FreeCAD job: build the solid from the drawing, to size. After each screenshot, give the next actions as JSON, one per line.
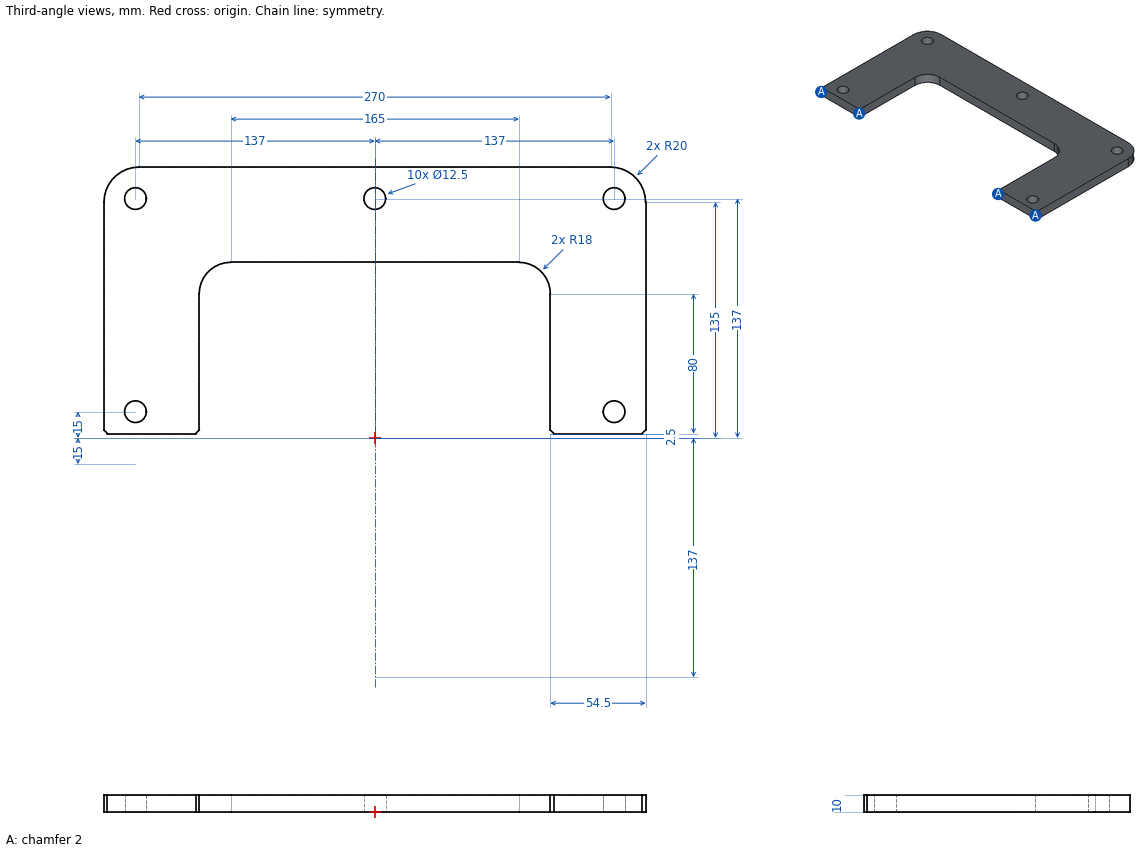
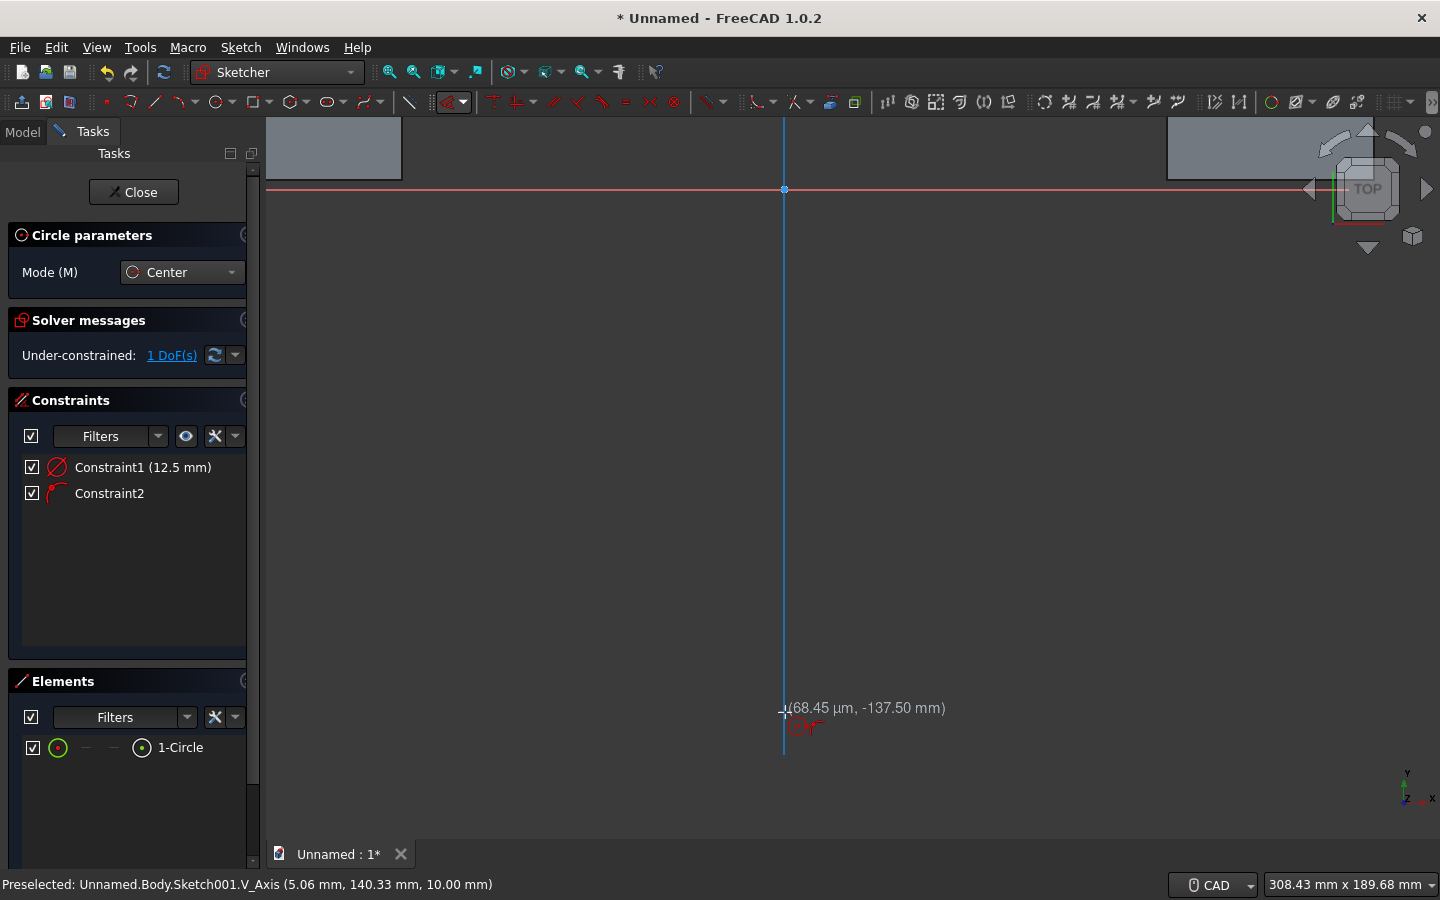
{"action": "left_click", "coordinate": [784, 711]}
{"action": "mouse_move", "coordinate": [801, 694]}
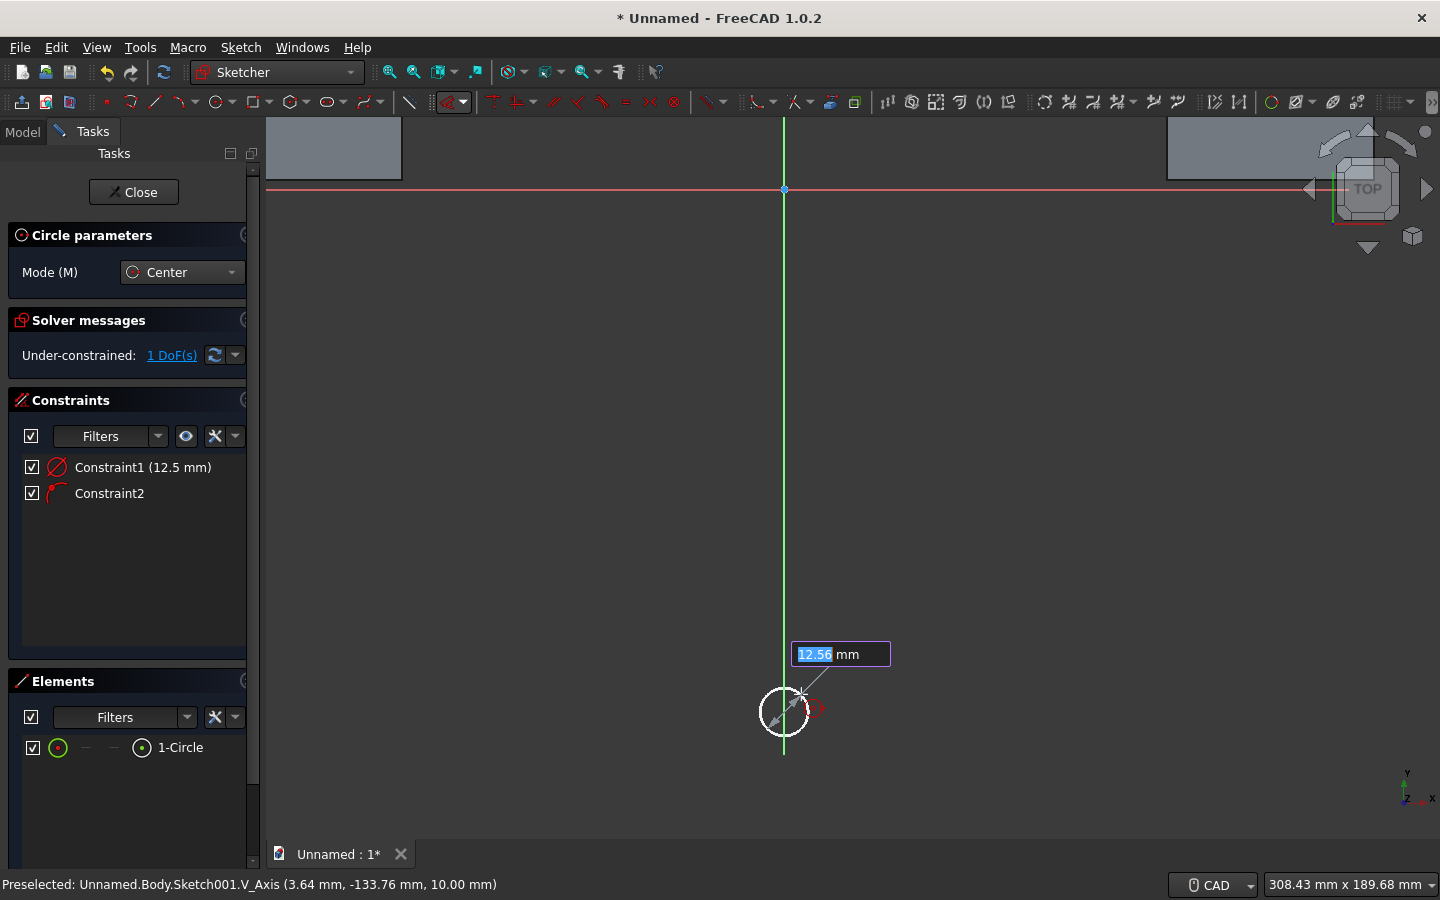
{"action": "type", "text": "12.5"}
{"action": "key", "text": "Return"}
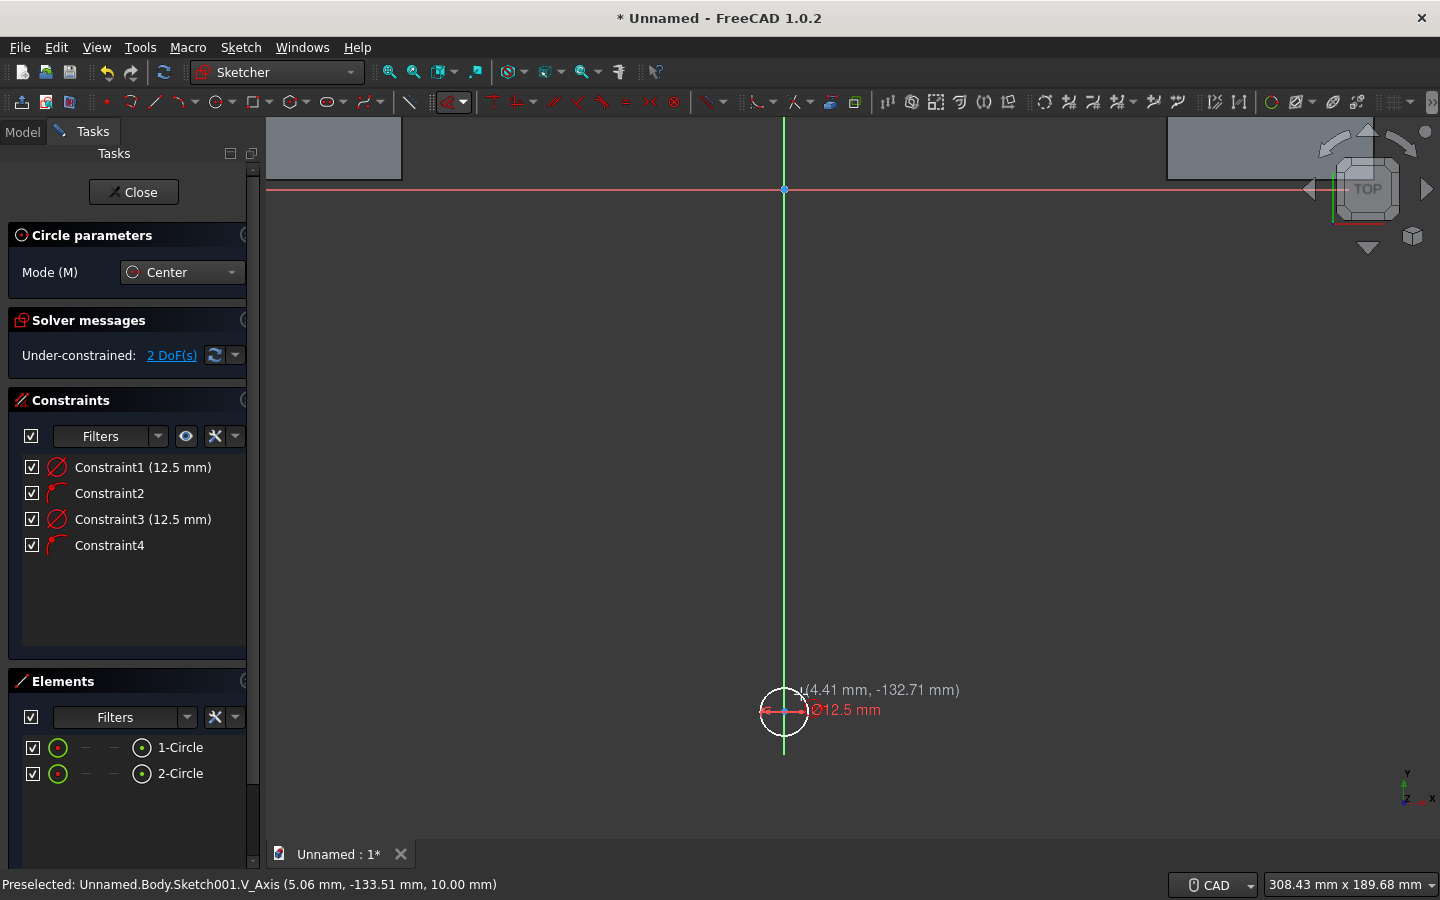
{"action": "scroll", "coordinate": [785, 713], "scroll_direction": "down", "scroll_amount": 4}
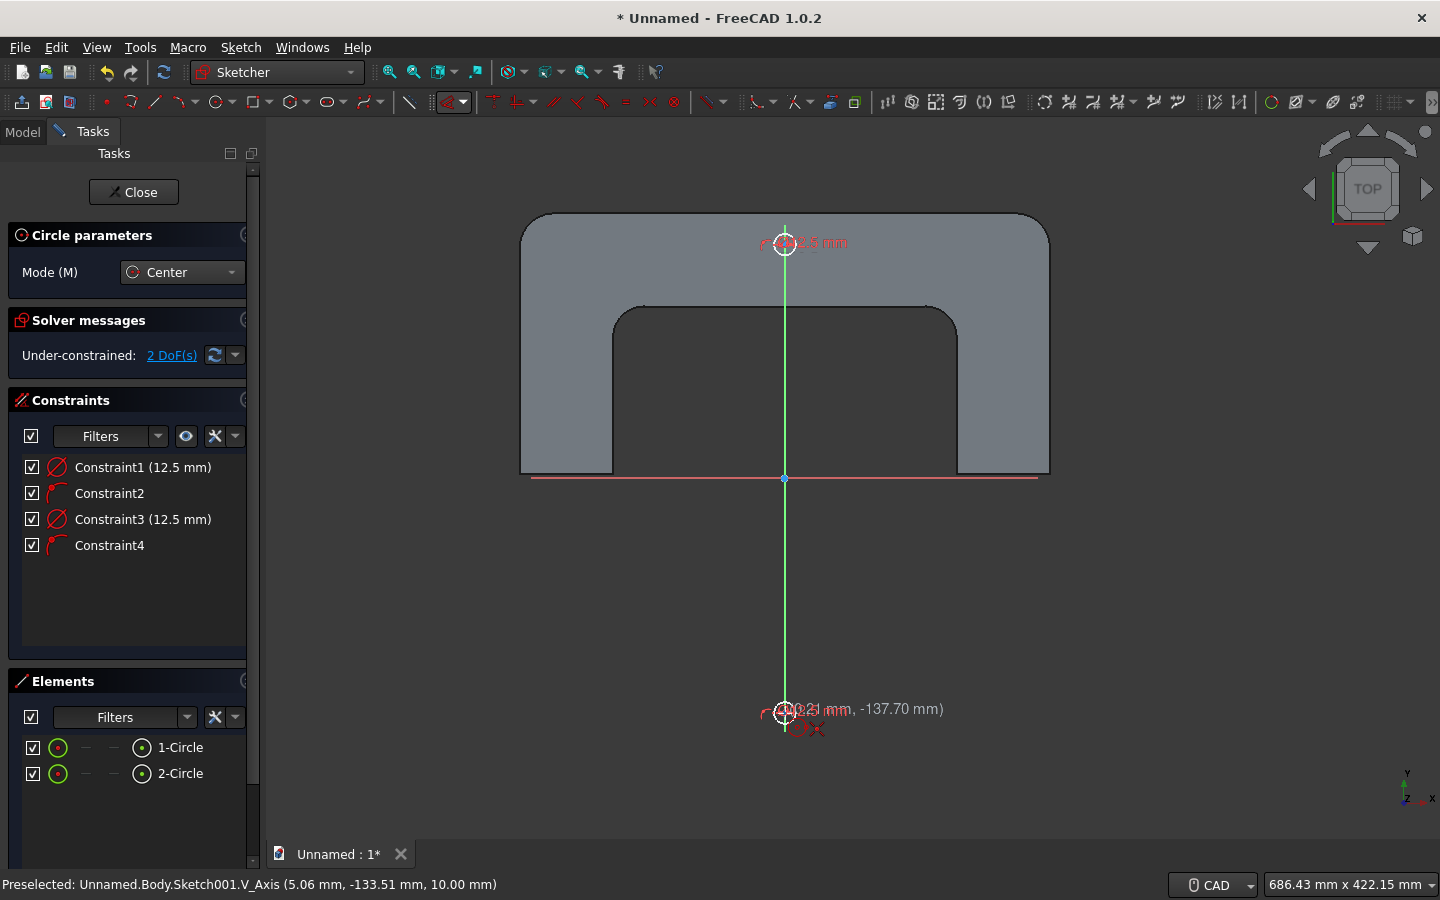
{"action": "scroll", "coordinate": [551, 244], "scroll_direction": "up", "scroll_amount": 4}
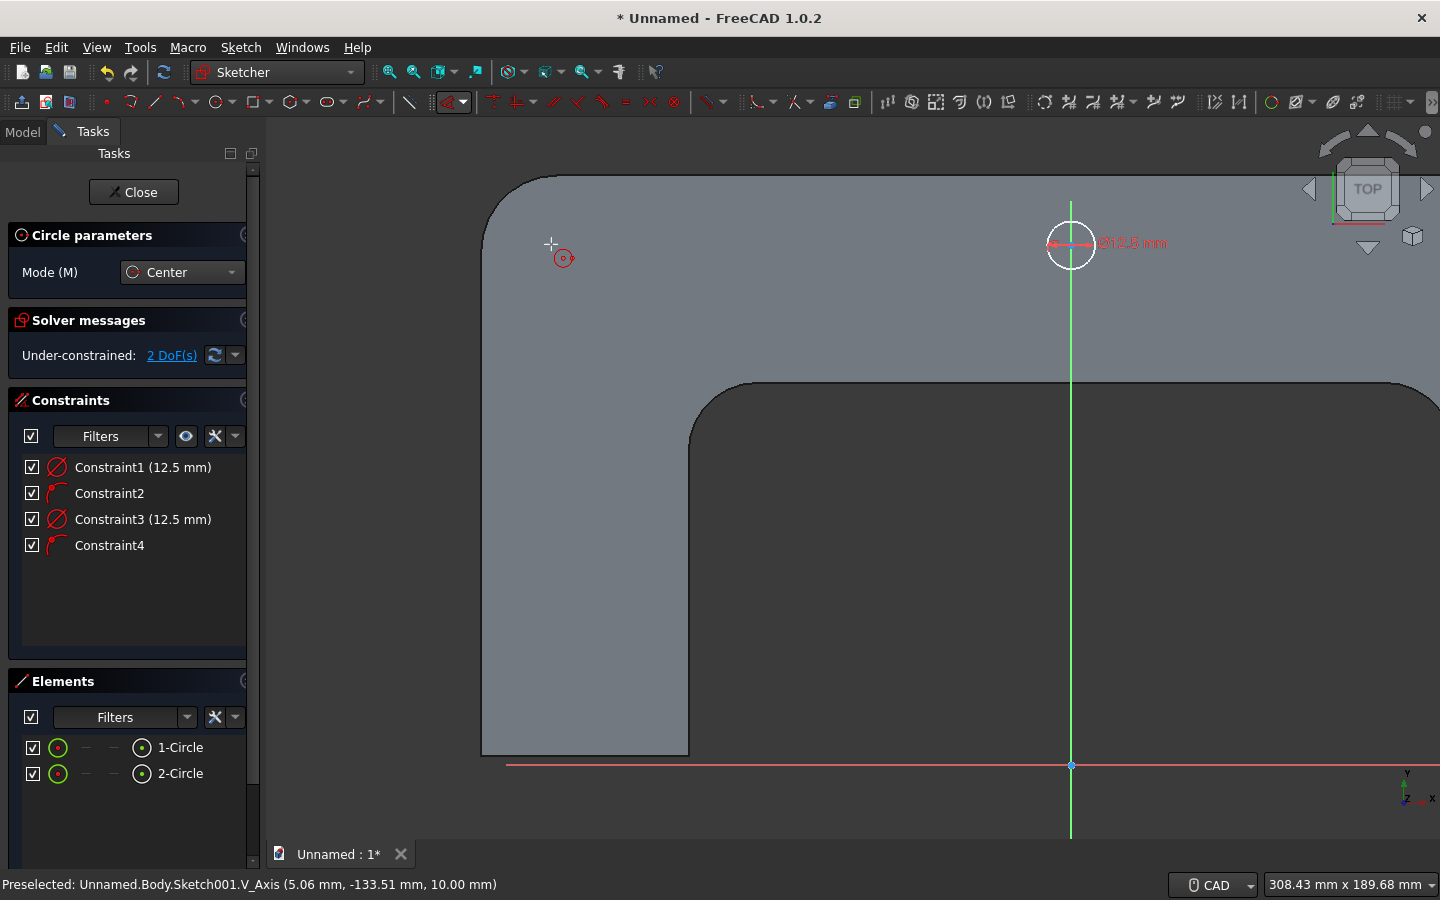
{"action": "left_click", "coordinate": [550, 244]}
{"action": "mouse_move", "coordinate": [567, 227]}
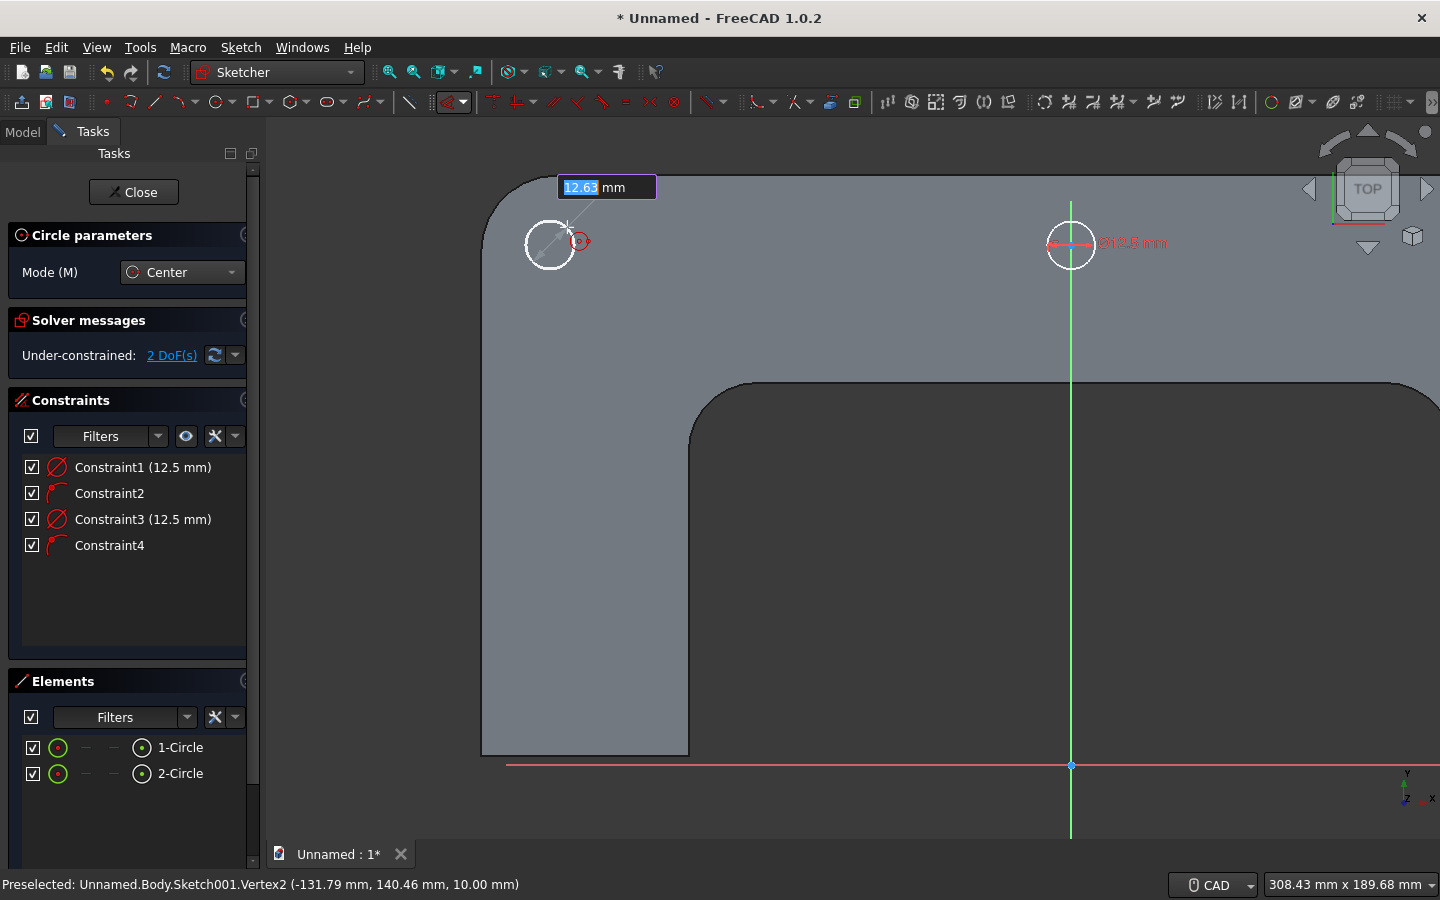
{"action": "type", "text": "12.5"}
{"action": "key", "text": "Return"}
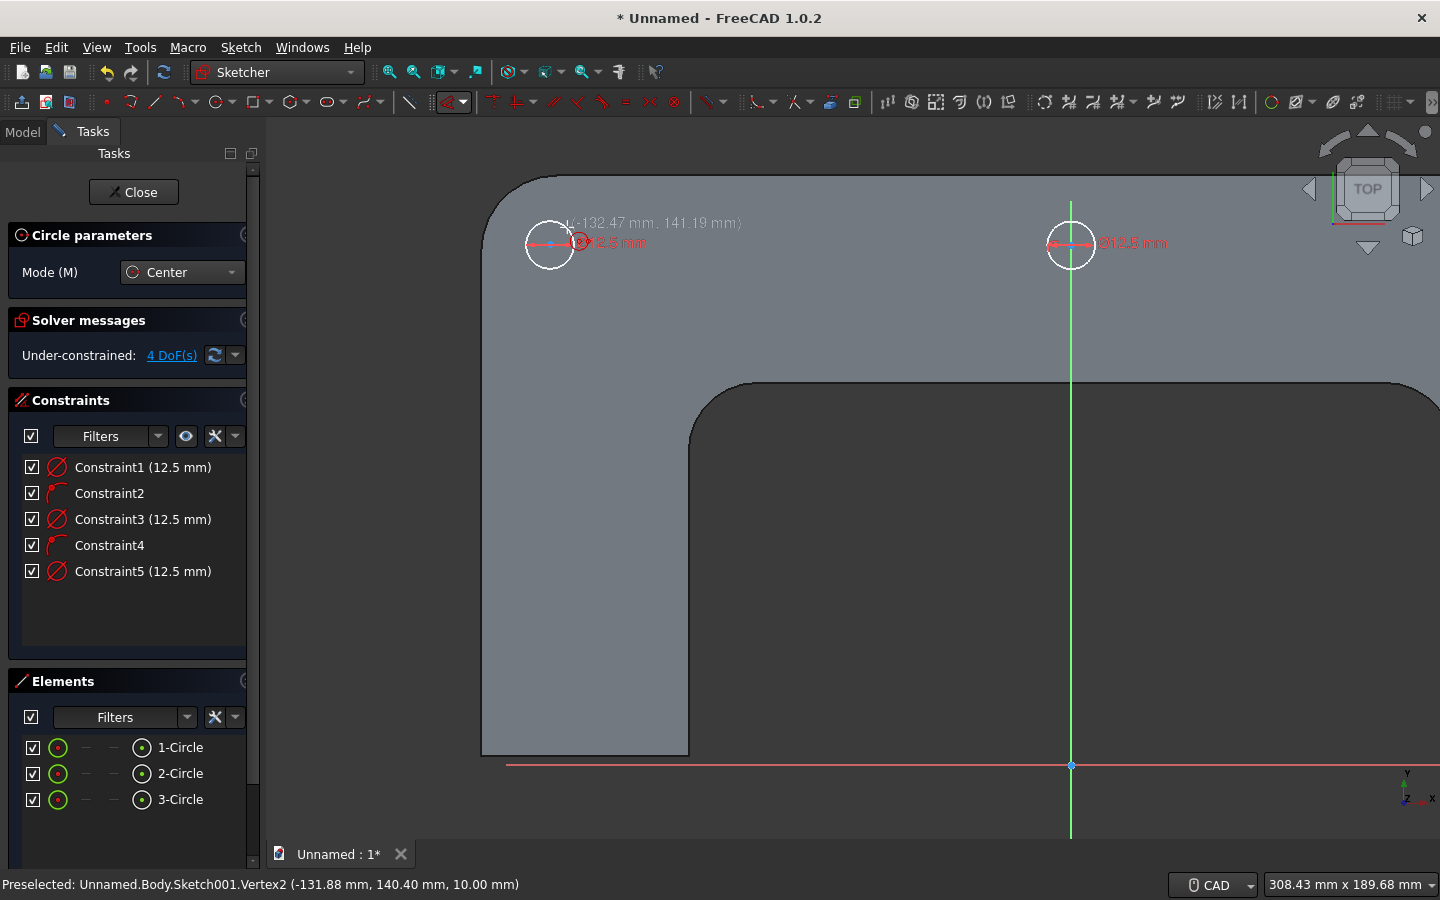
{"action": "scroll", "coordinate": [551, 243], "scroll_direction": "down", "scroll_amount": 4}